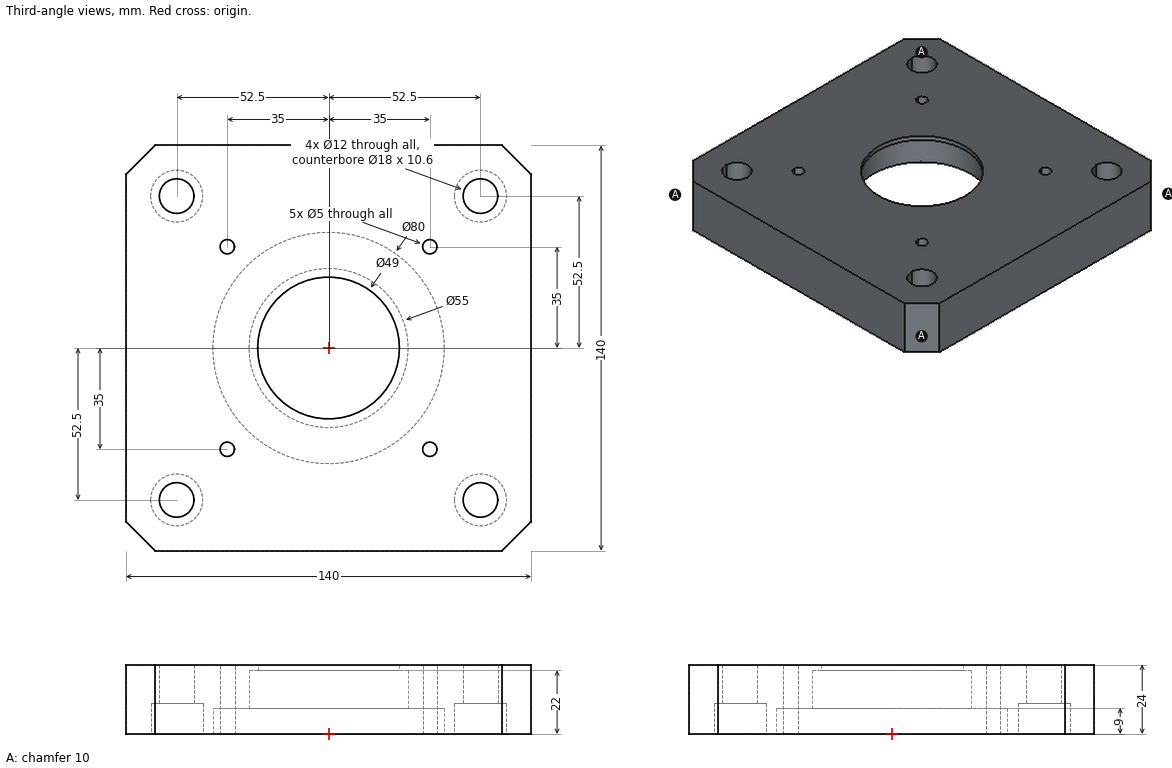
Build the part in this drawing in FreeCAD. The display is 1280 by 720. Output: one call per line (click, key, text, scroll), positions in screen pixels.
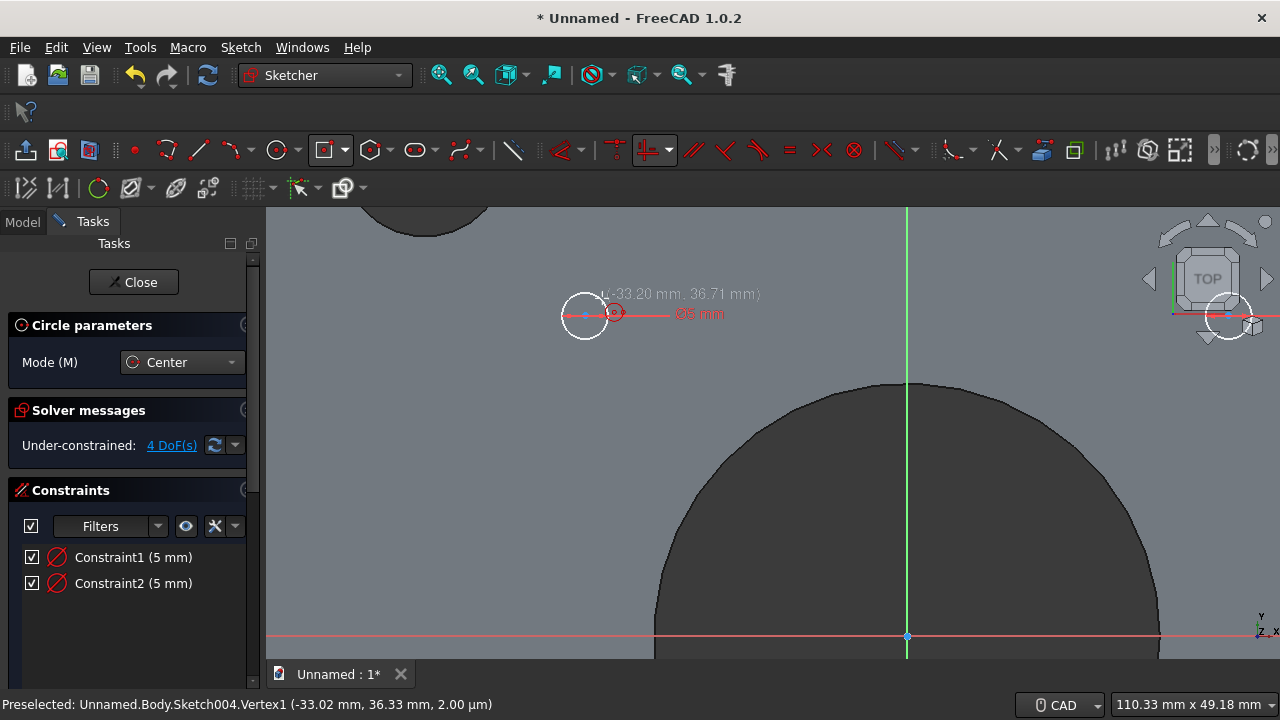
scroll(587, 315, down, 5)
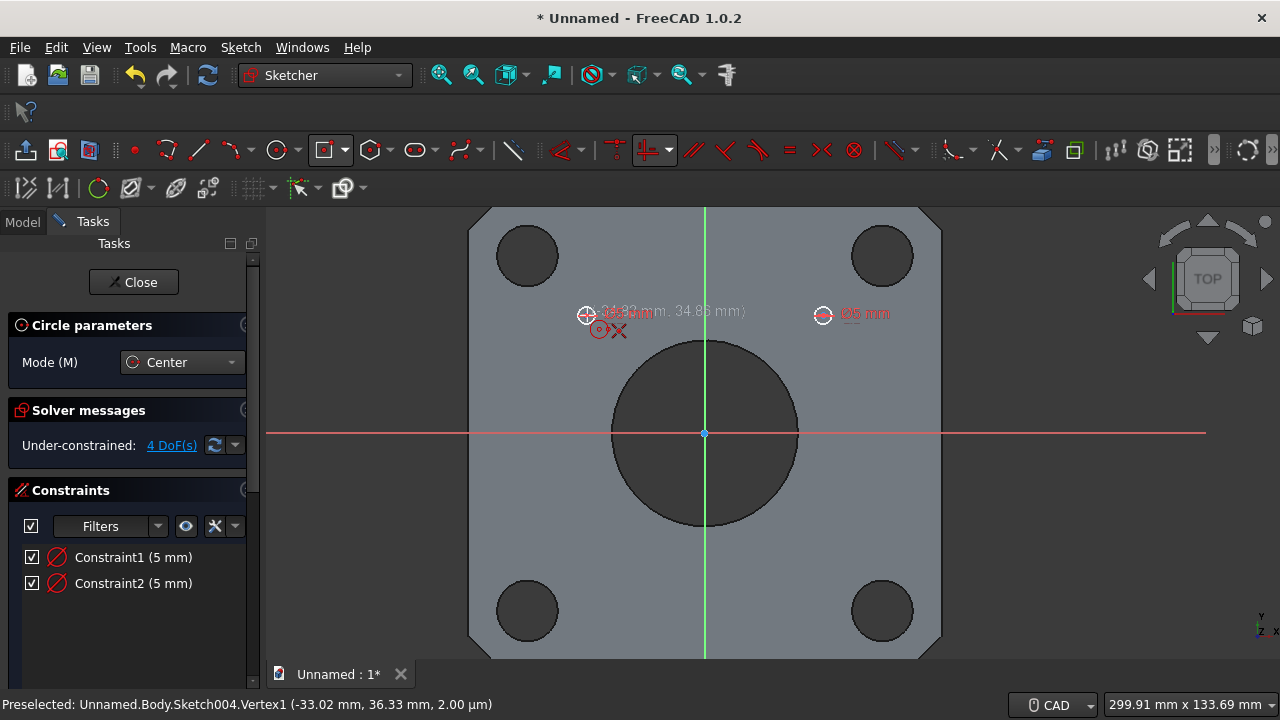
scroll(587, 552, up, 5)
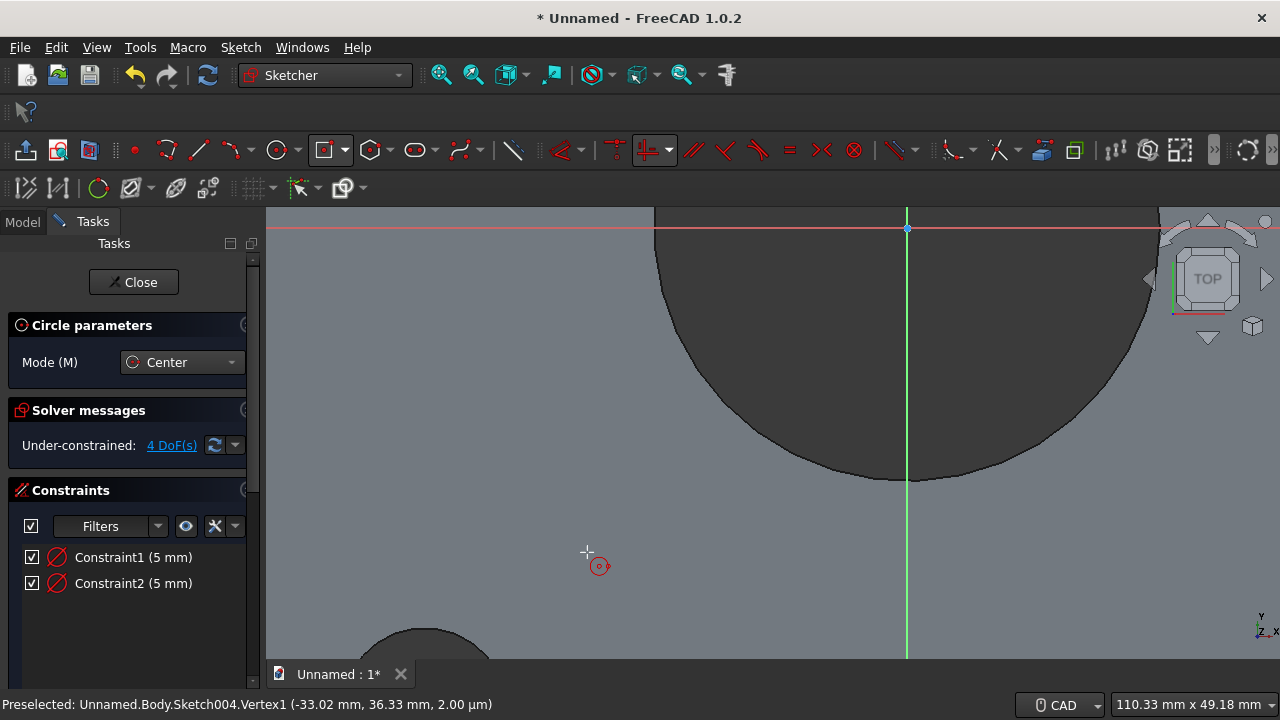
click(585, 550)
move(602, 534)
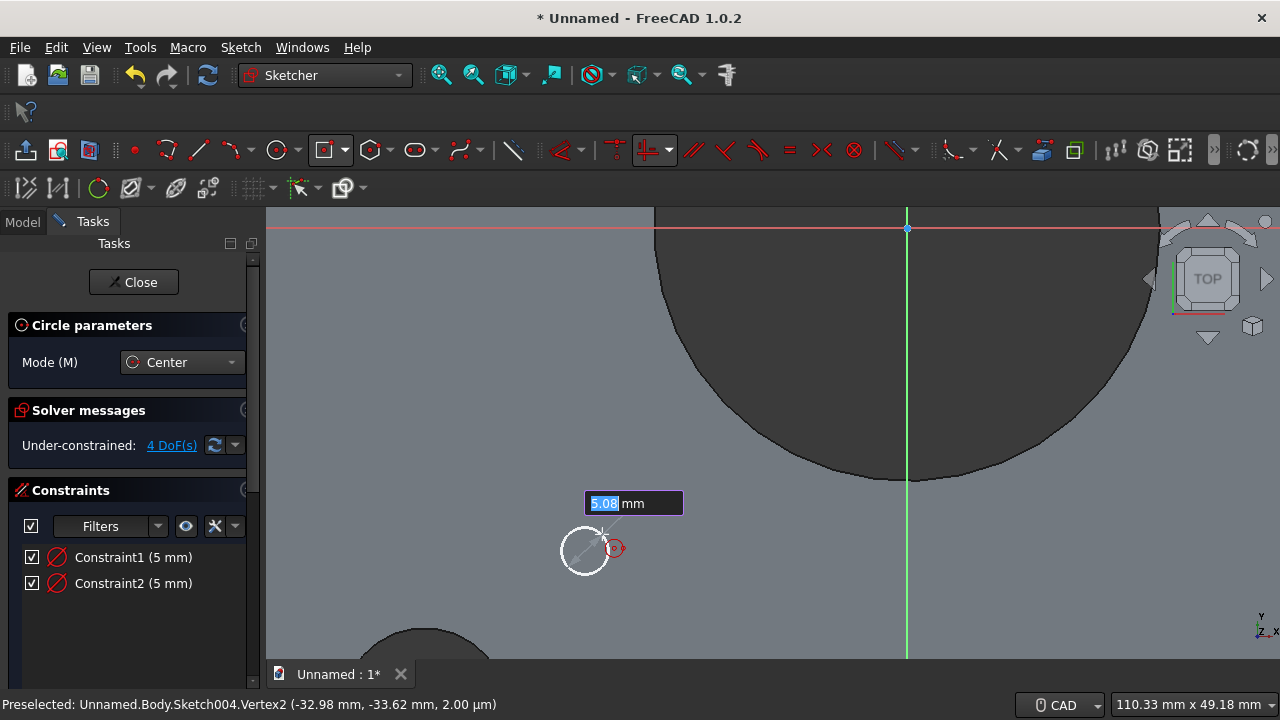
text(5)
key(Return)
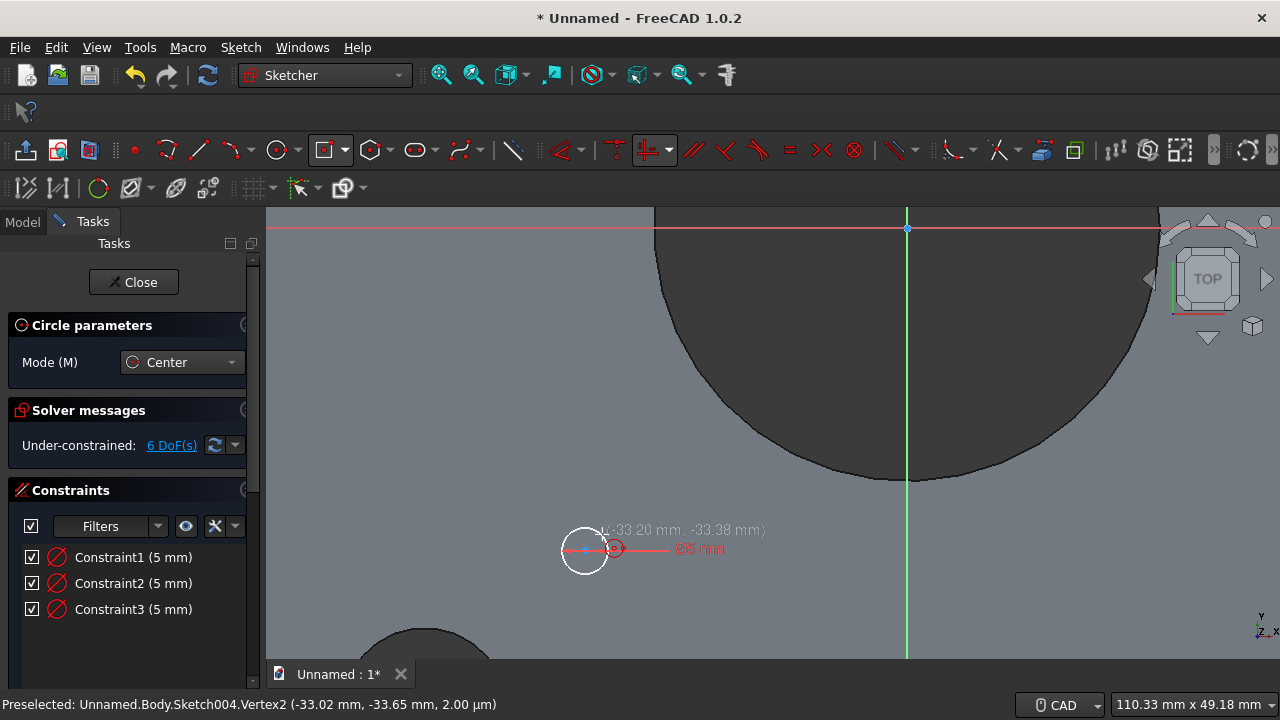
scroll(587, 552, down, 5)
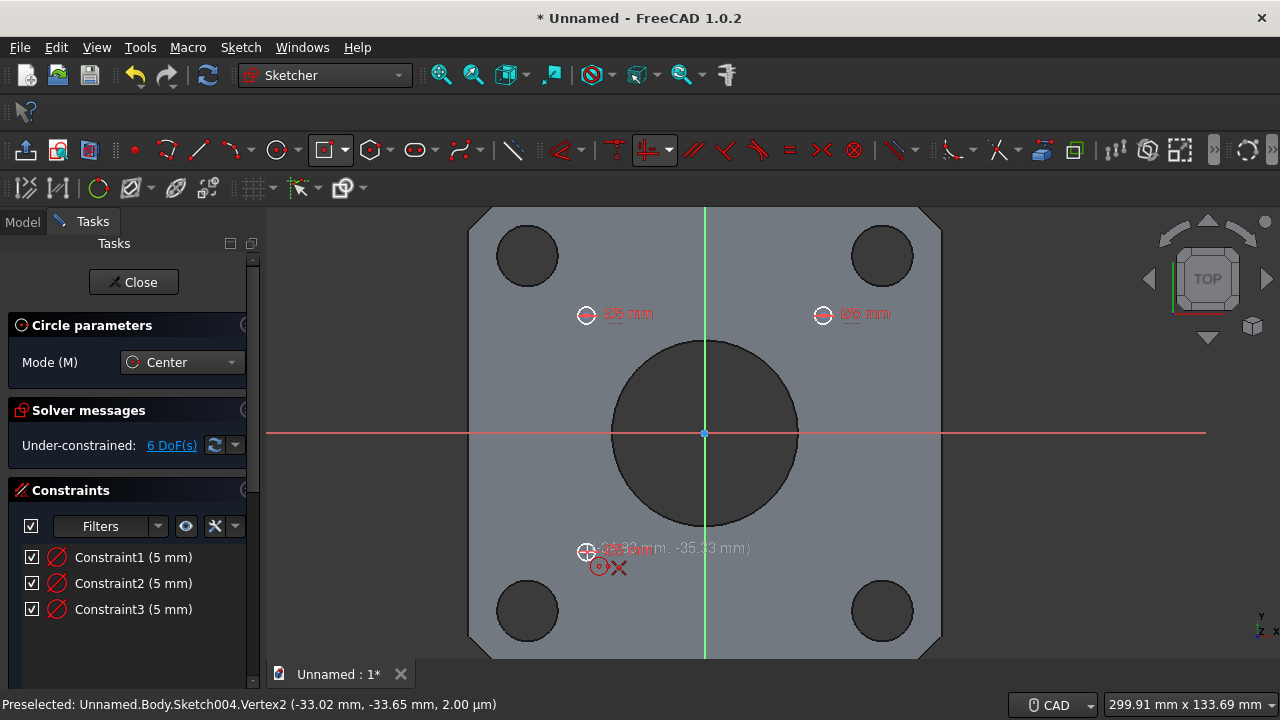
scroll(823, 552, up, 5)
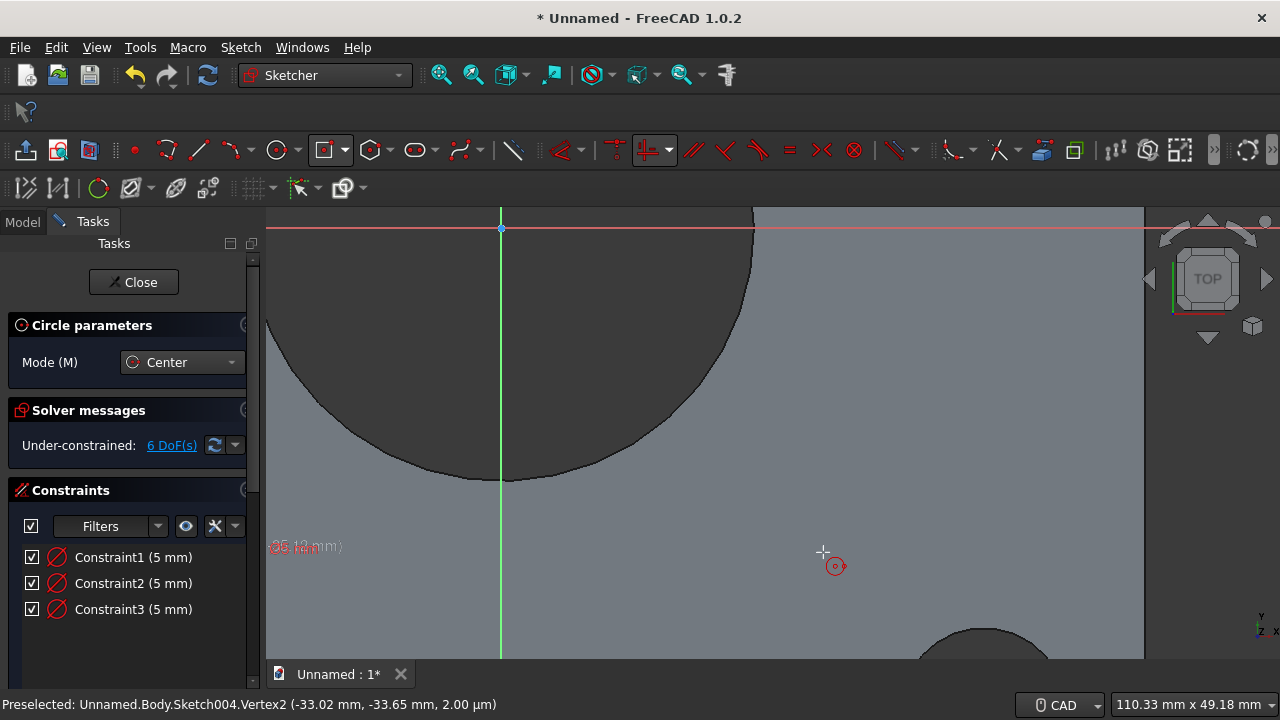
click(823, 550)
move(839, 534)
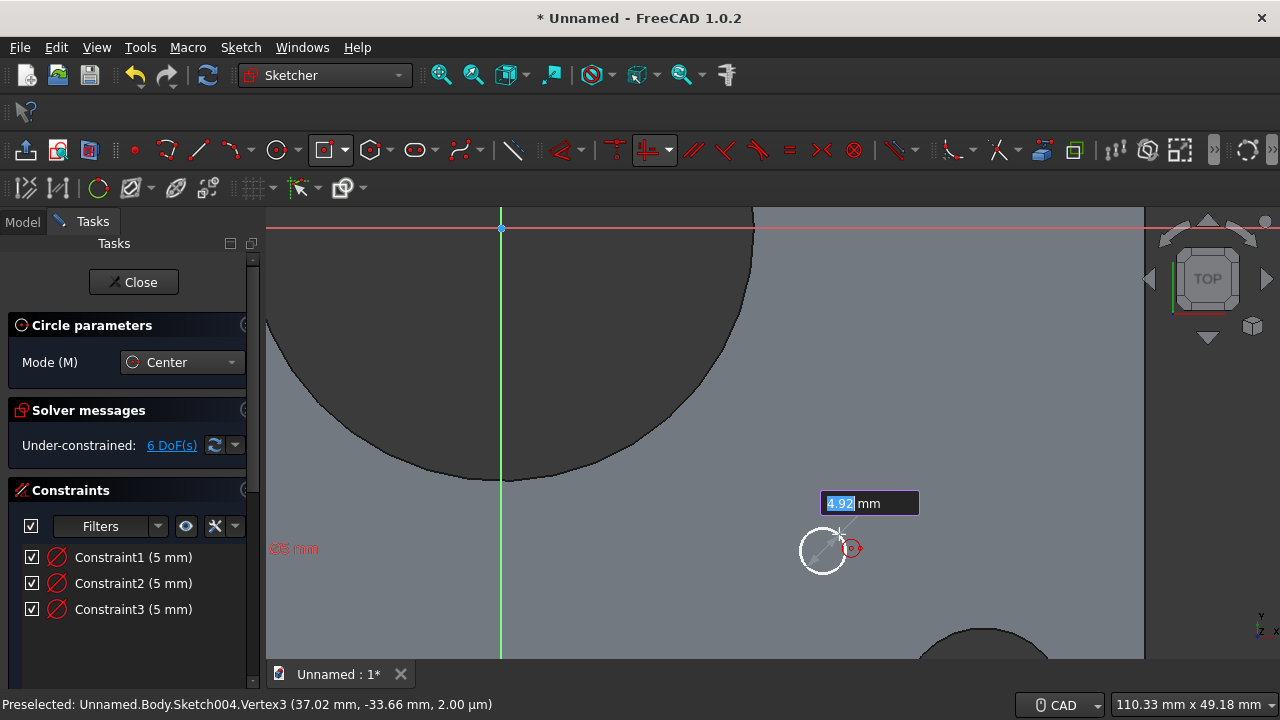
text(5)
key(Return)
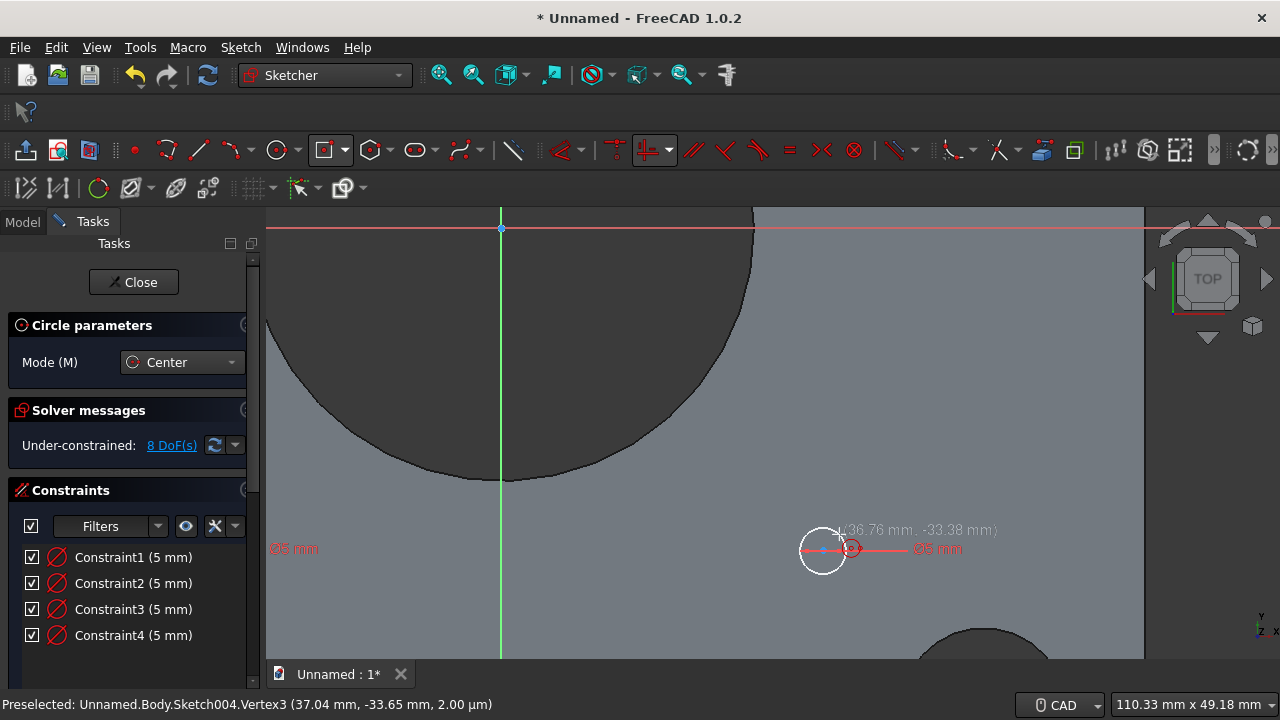
scroll(823, 552, down, 5)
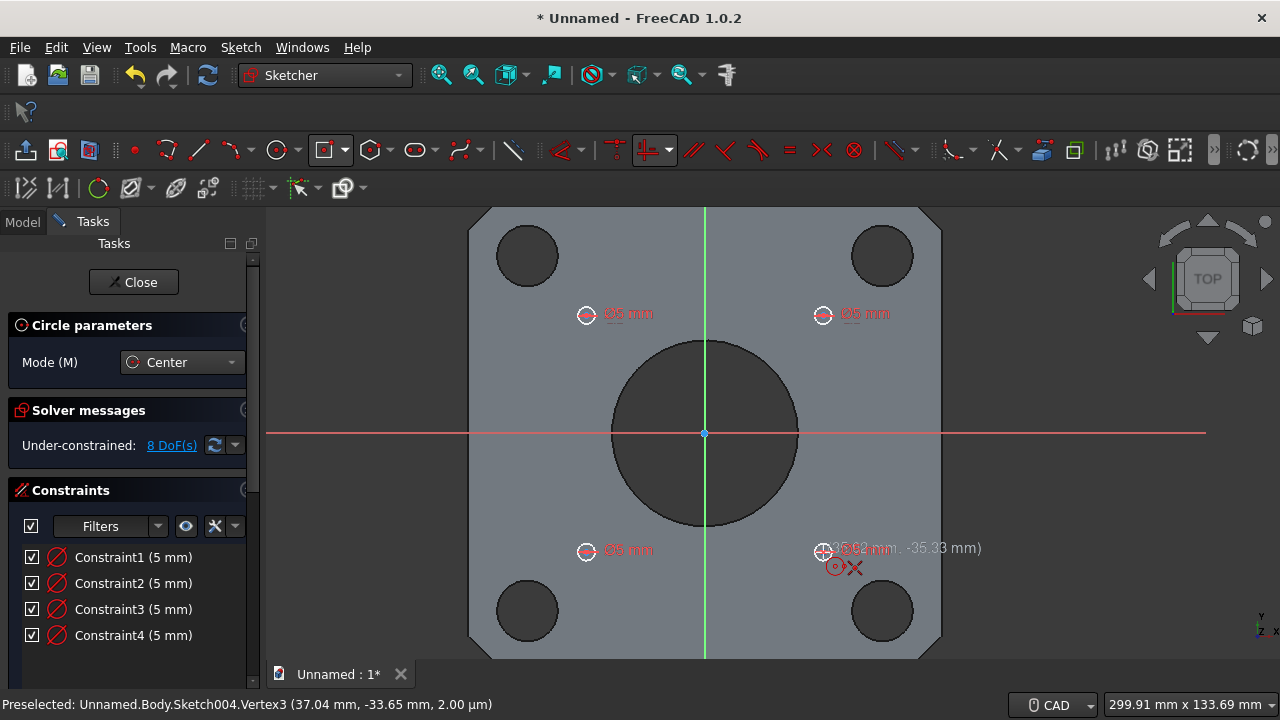
scroll(705, 433, up, 5)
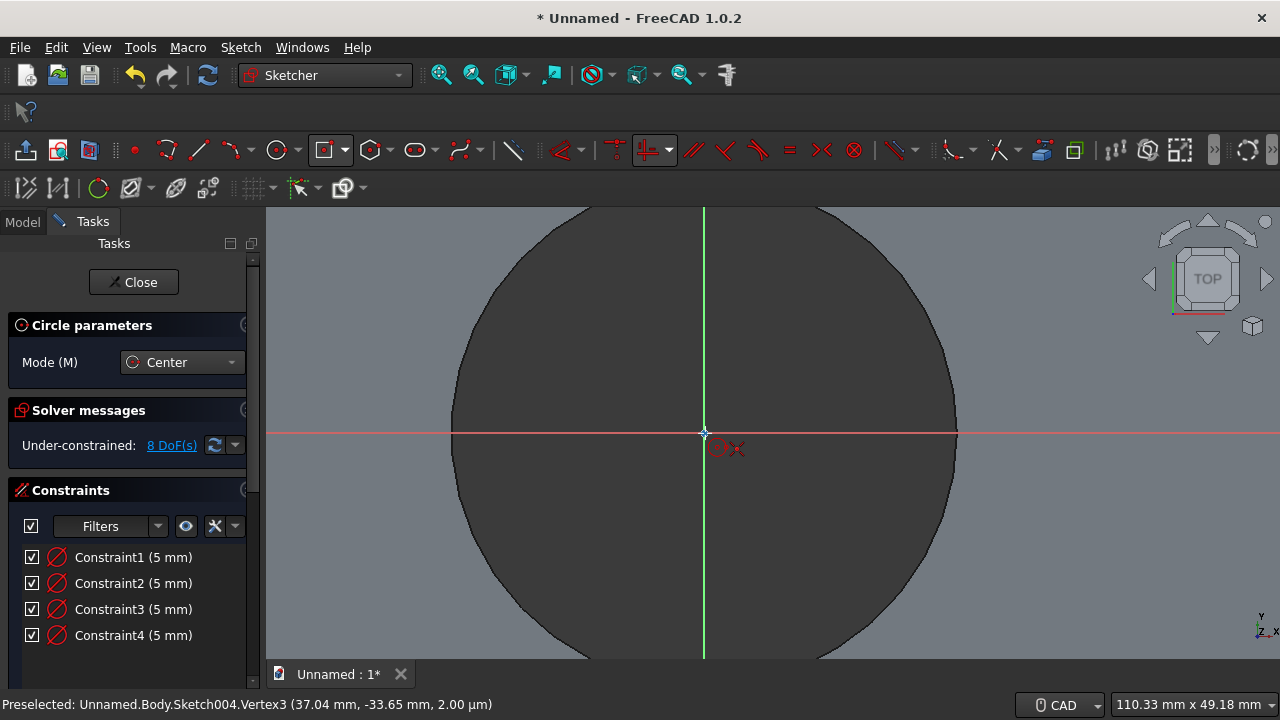
click(704, 433)
move(720, 417)